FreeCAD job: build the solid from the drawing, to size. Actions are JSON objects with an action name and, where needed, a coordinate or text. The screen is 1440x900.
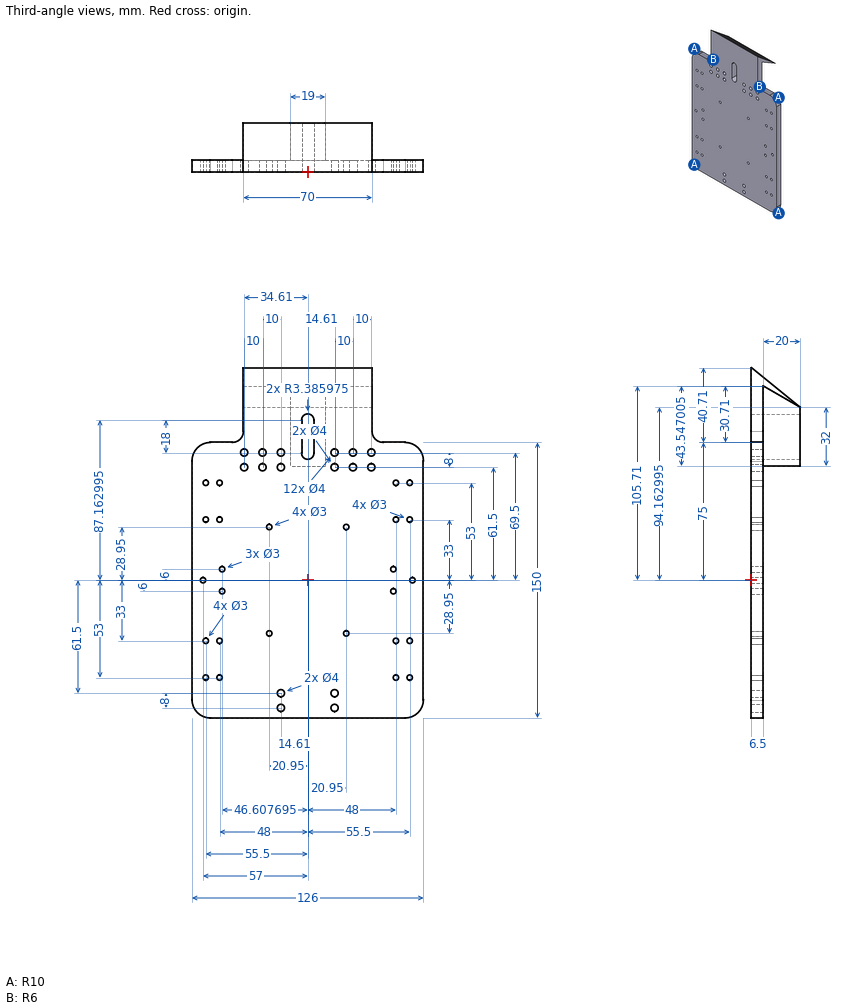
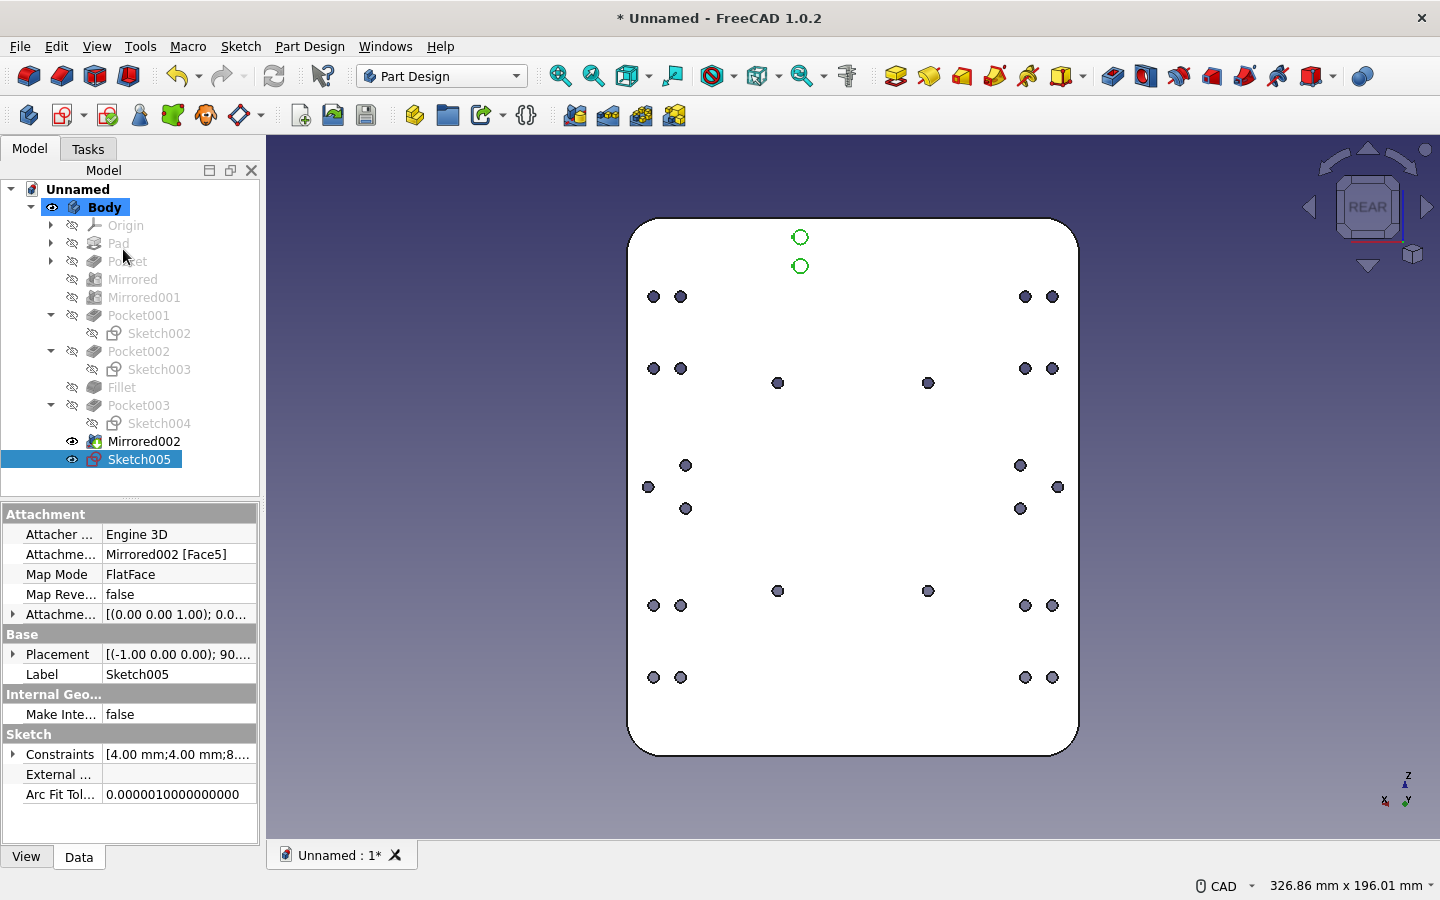
{"action": "left_click", "coordinate": [1113, 76]}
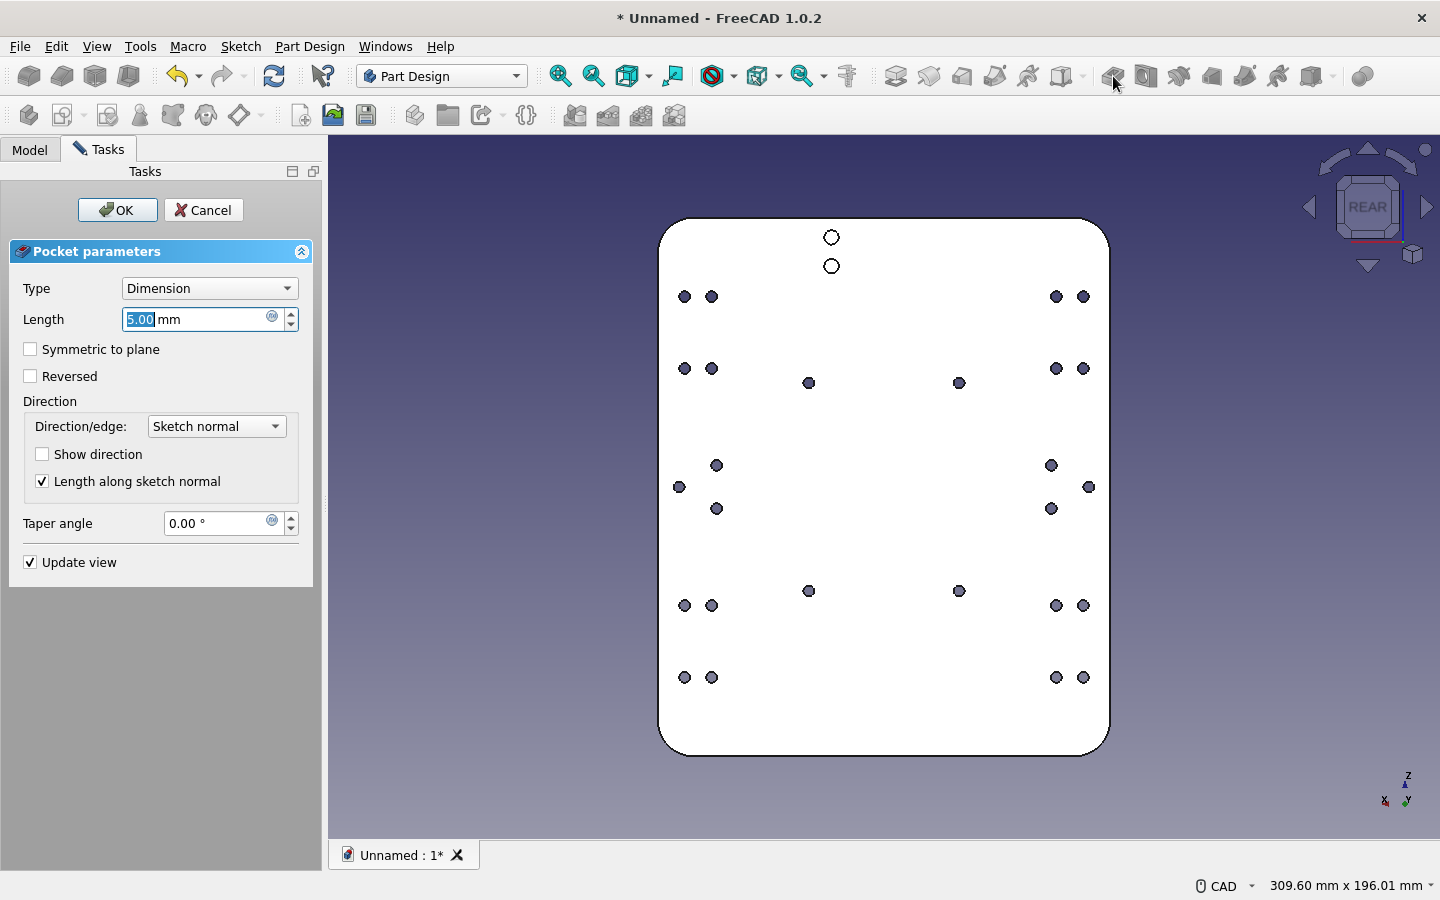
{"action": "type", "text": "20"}
{"action": "key", "text": "Tab"}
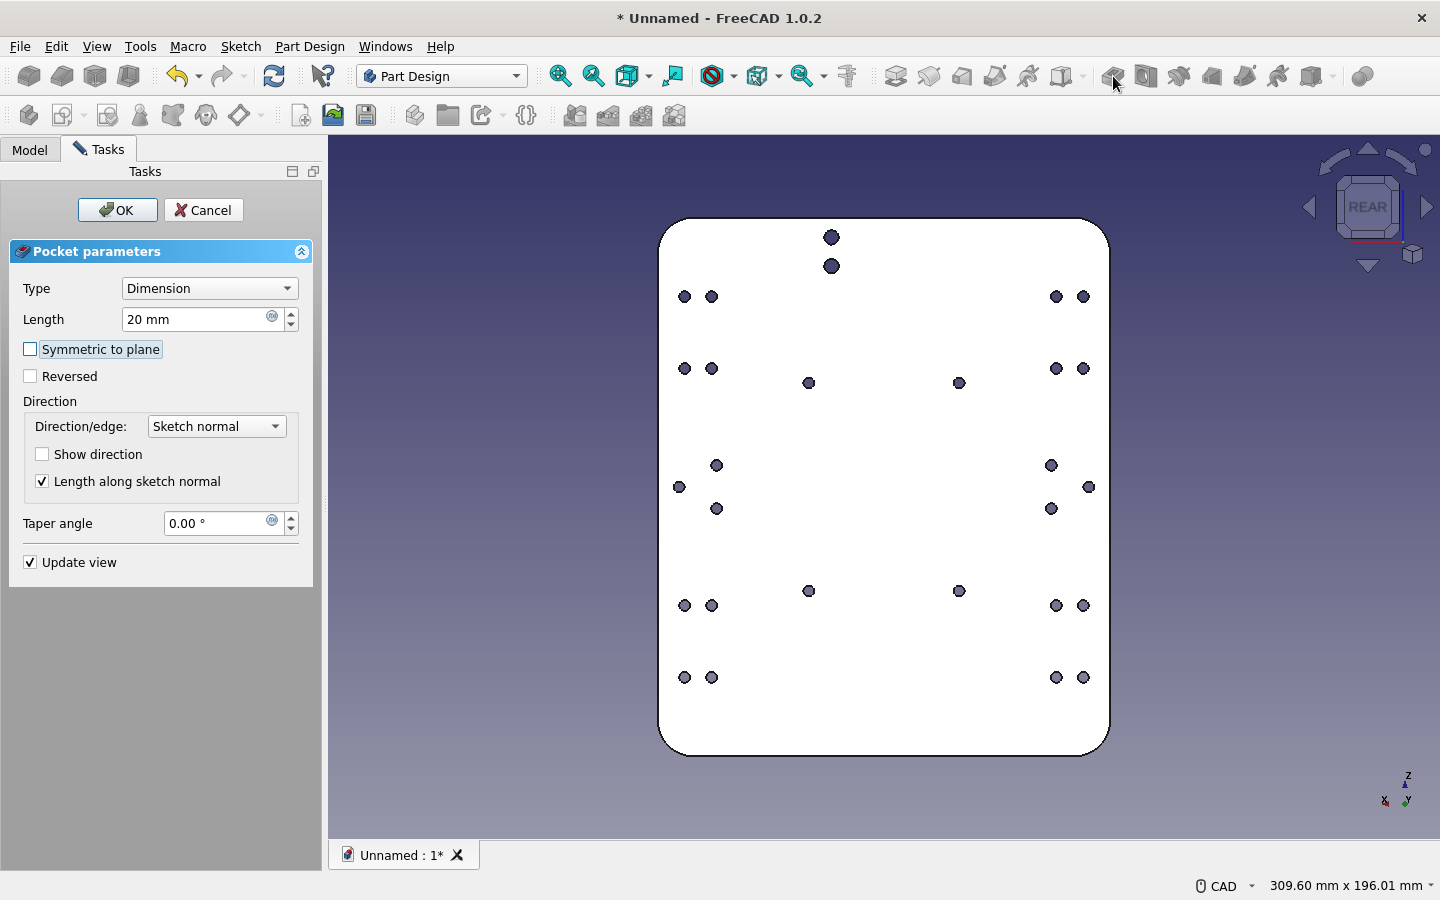
{"action": "left_click", "coordinate": [118, 210]}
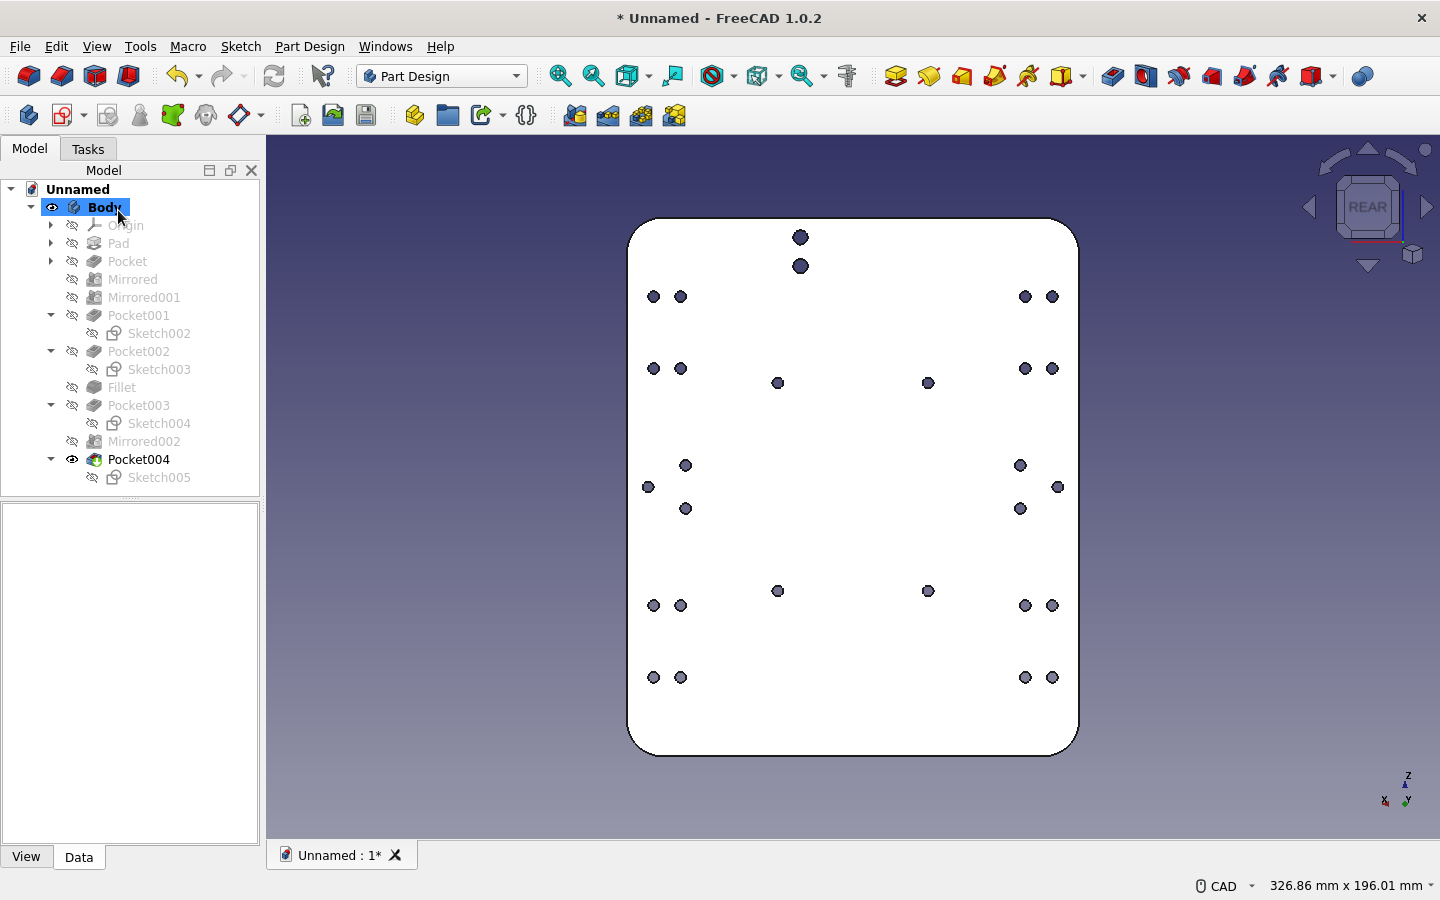
{"action": "left_click", "coordinate": [117, 459]}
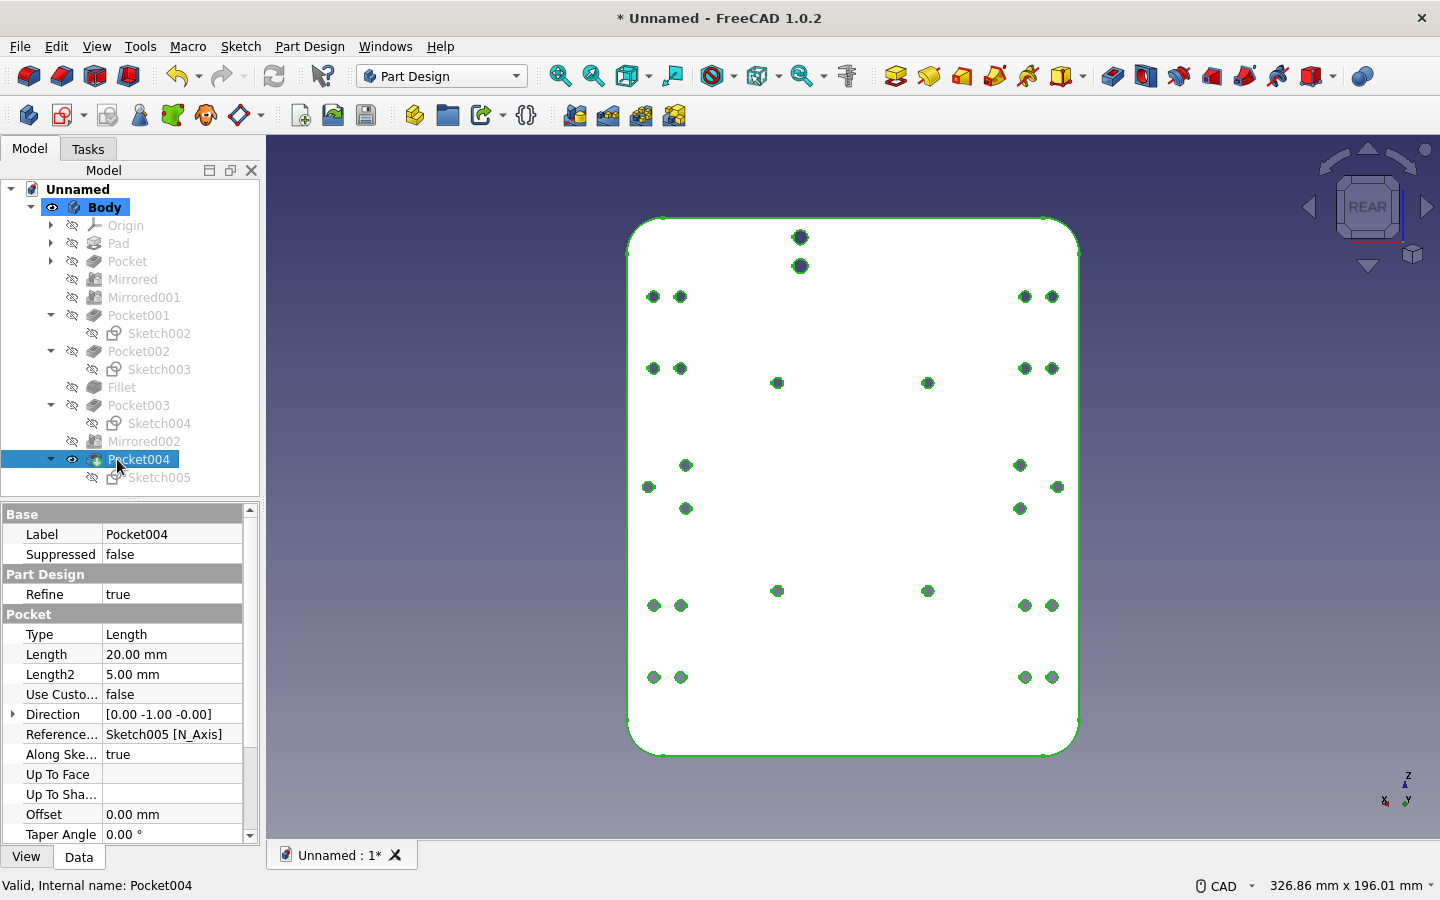
{"action": "left_click", "coordinate": [575, 116]}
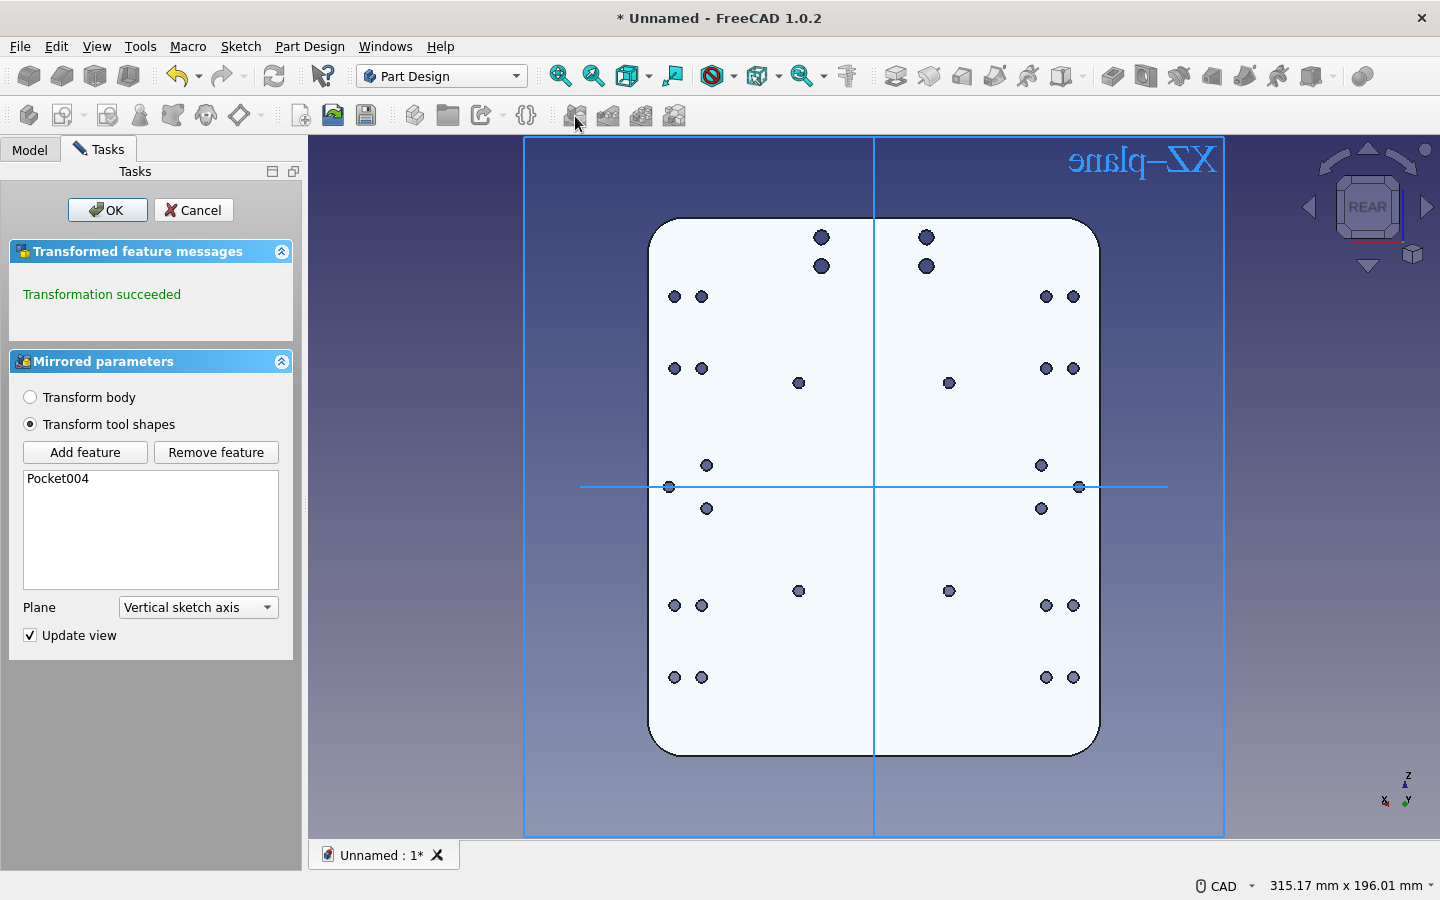
{"action": "left_click", "coordinate": [199, 608]}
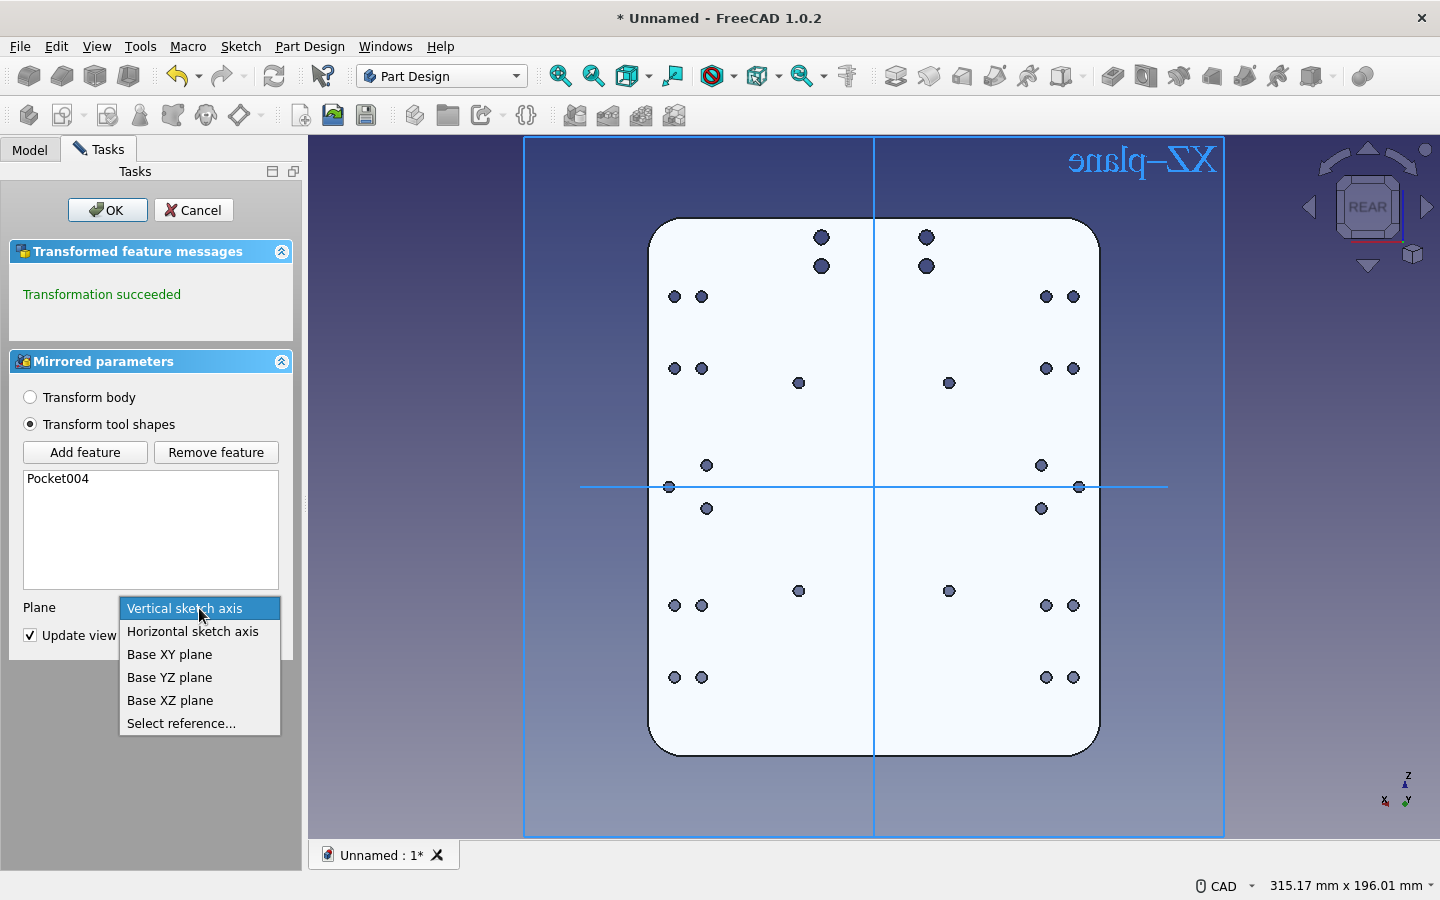
{"action": "left_click", "coordinate": [198, 678]}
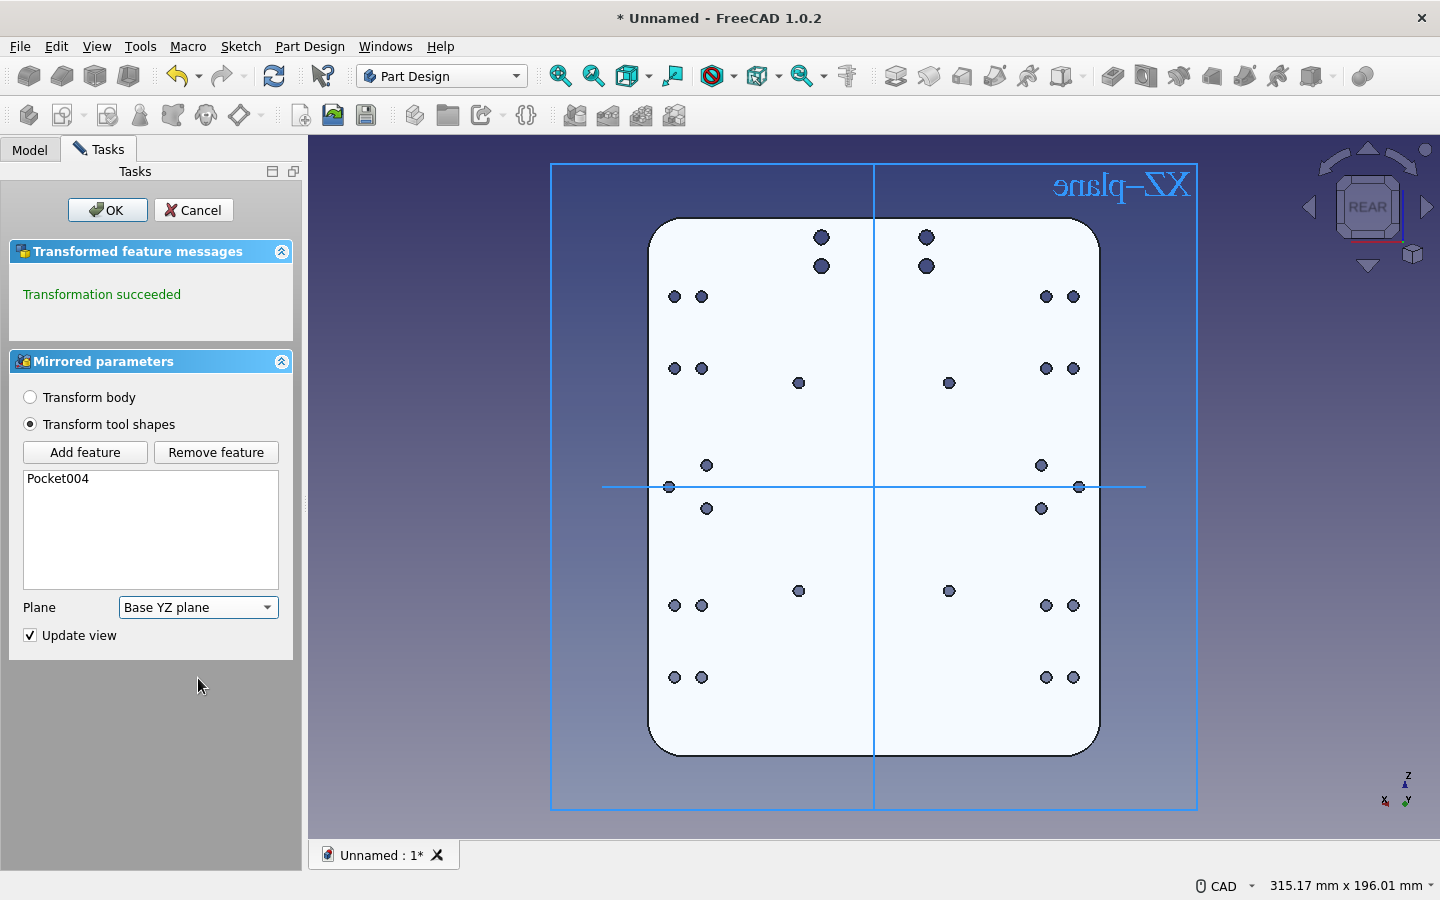
{"action": "left_click", "coordinate": [108, 210]}